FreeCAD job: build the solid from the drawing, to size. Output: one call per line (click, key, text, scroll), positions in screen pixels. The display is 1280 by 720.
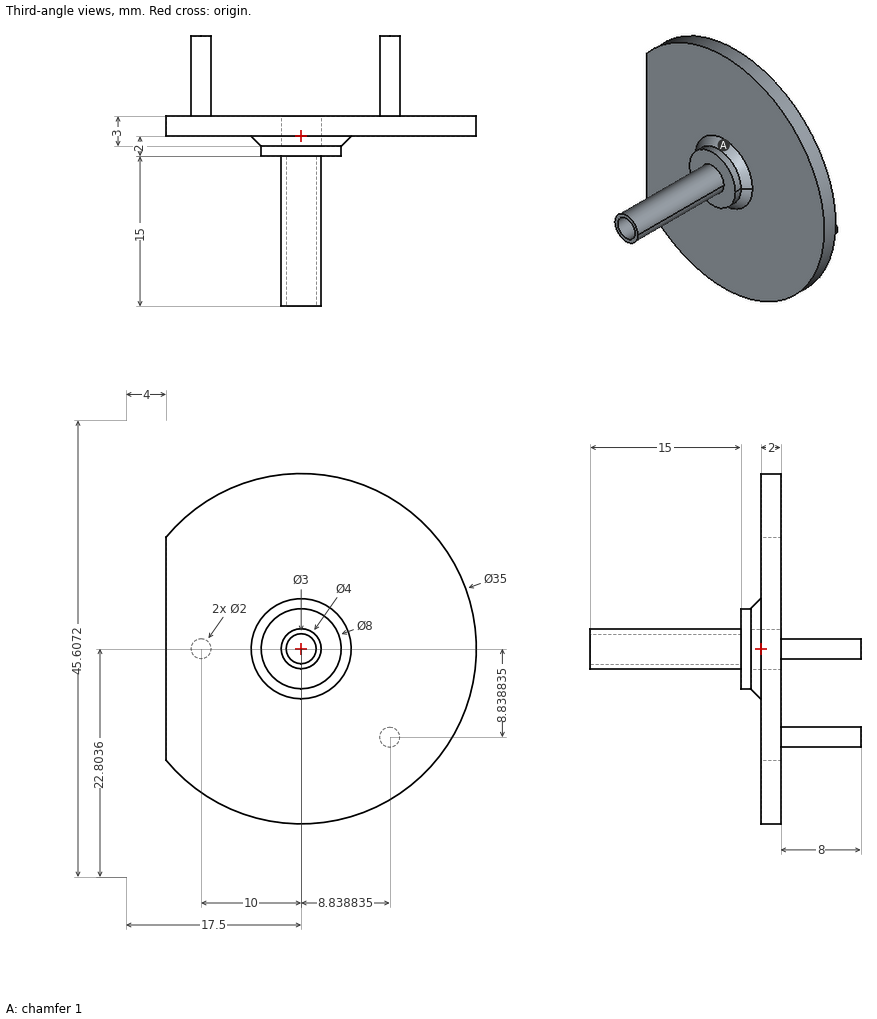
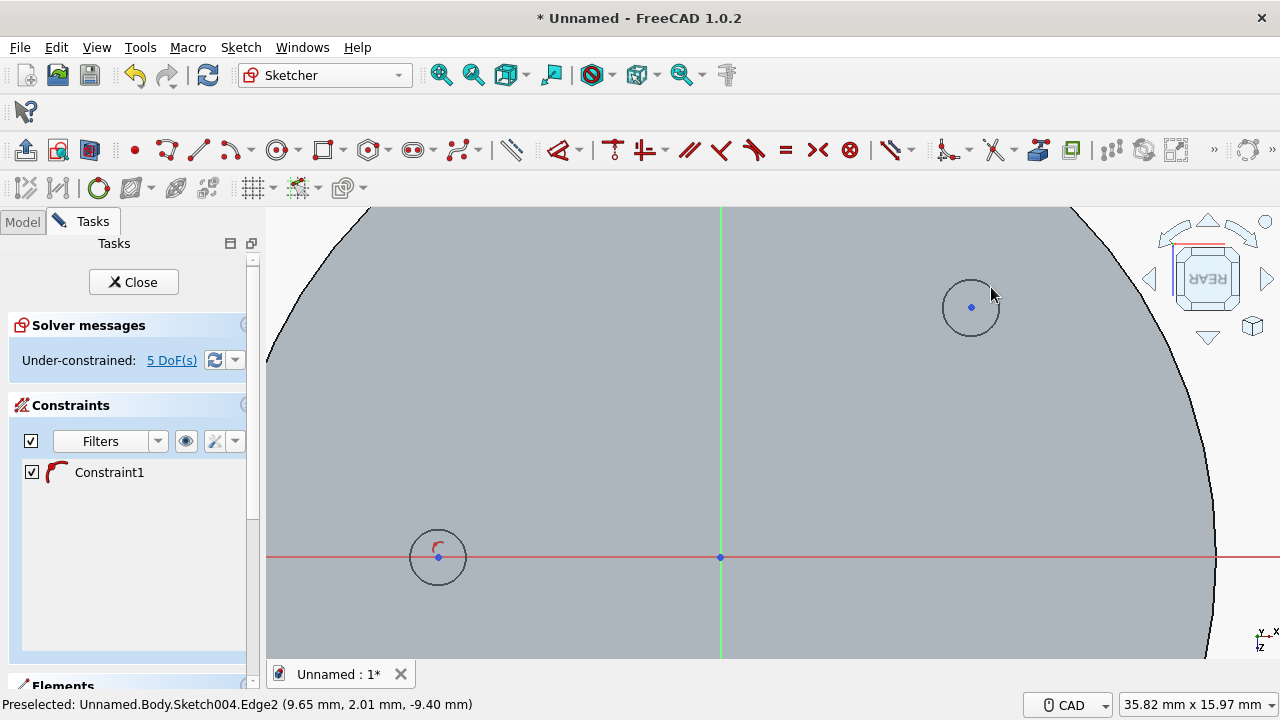
click(458, 538)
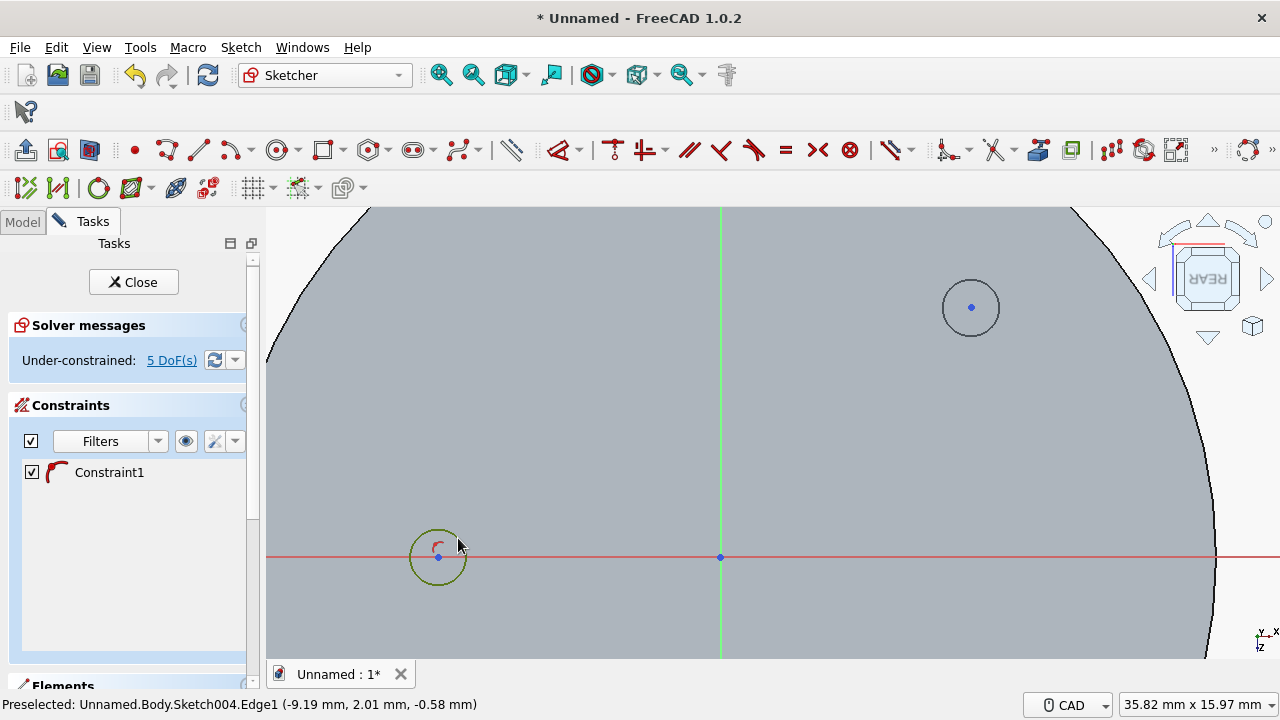
click(991, 288)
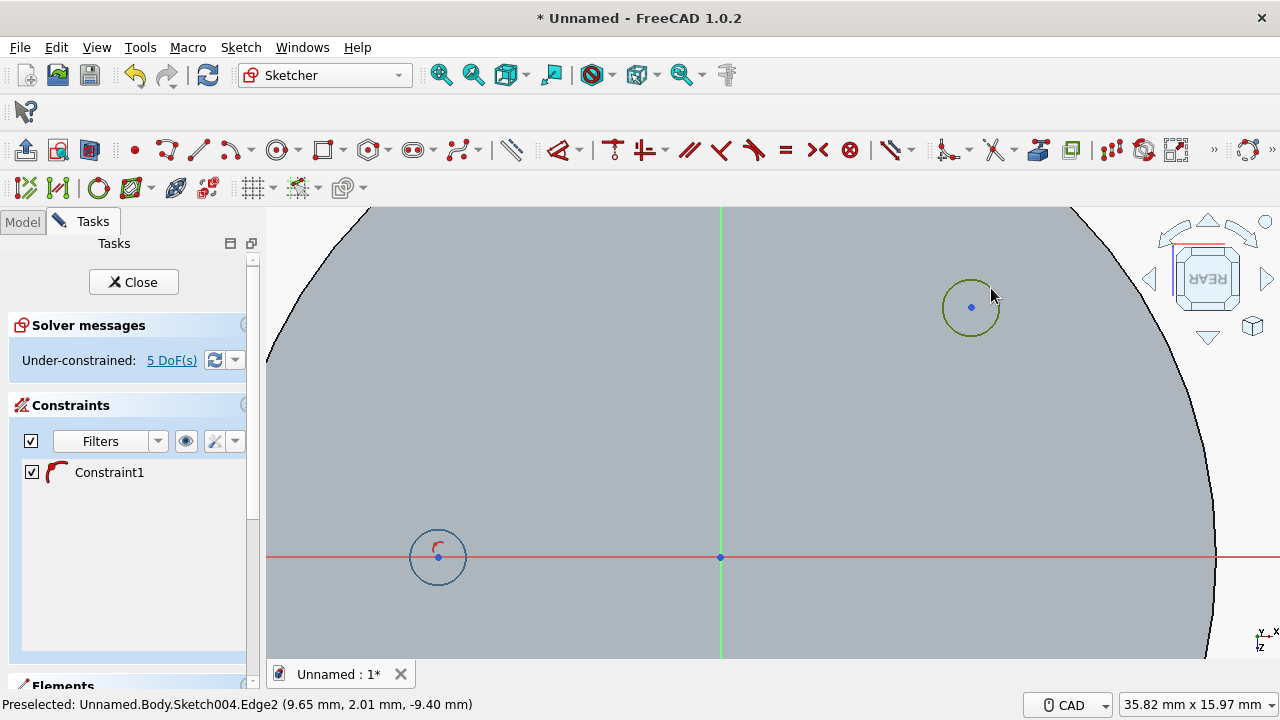
click(786, 150)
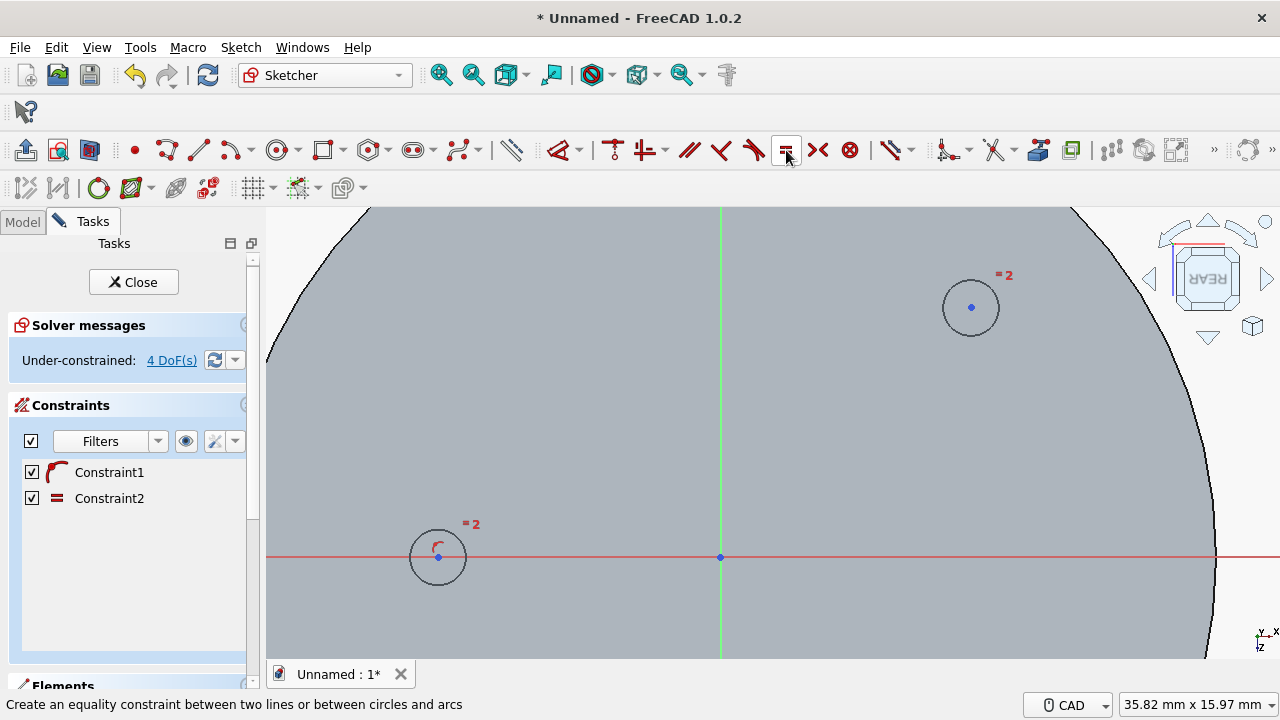
click(558, 150)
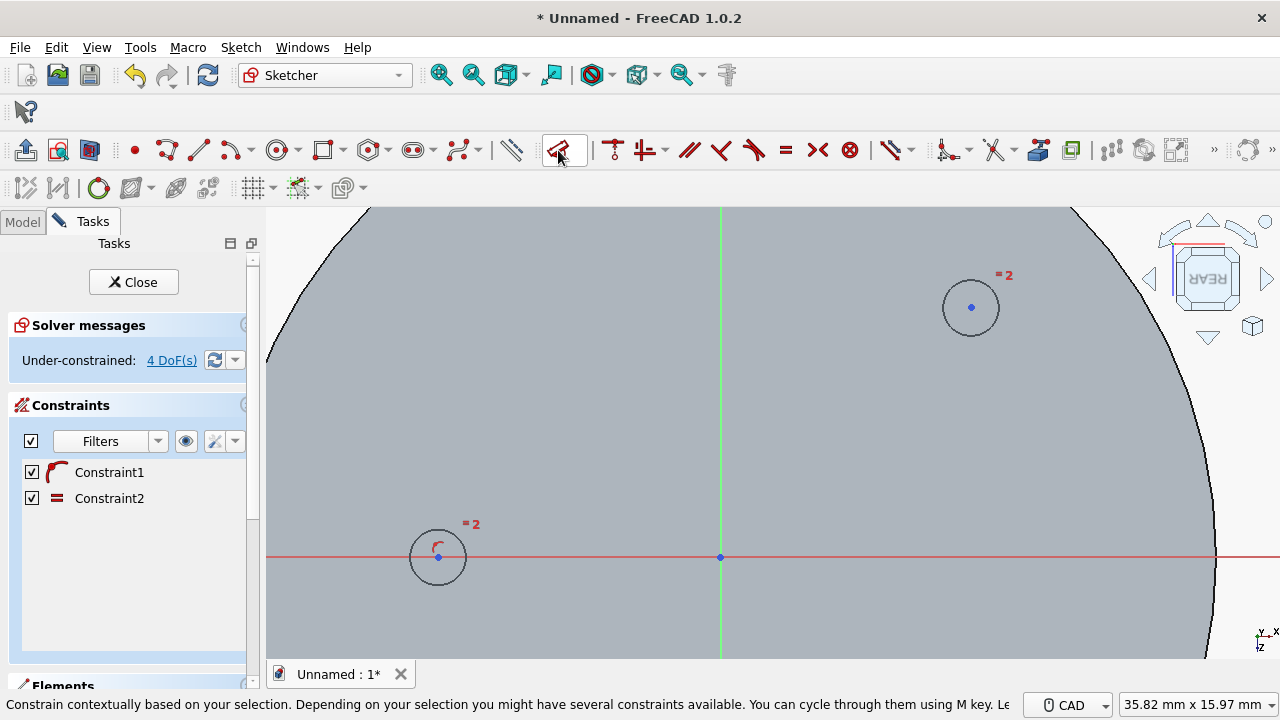
click(458, 538)
click(481, 516)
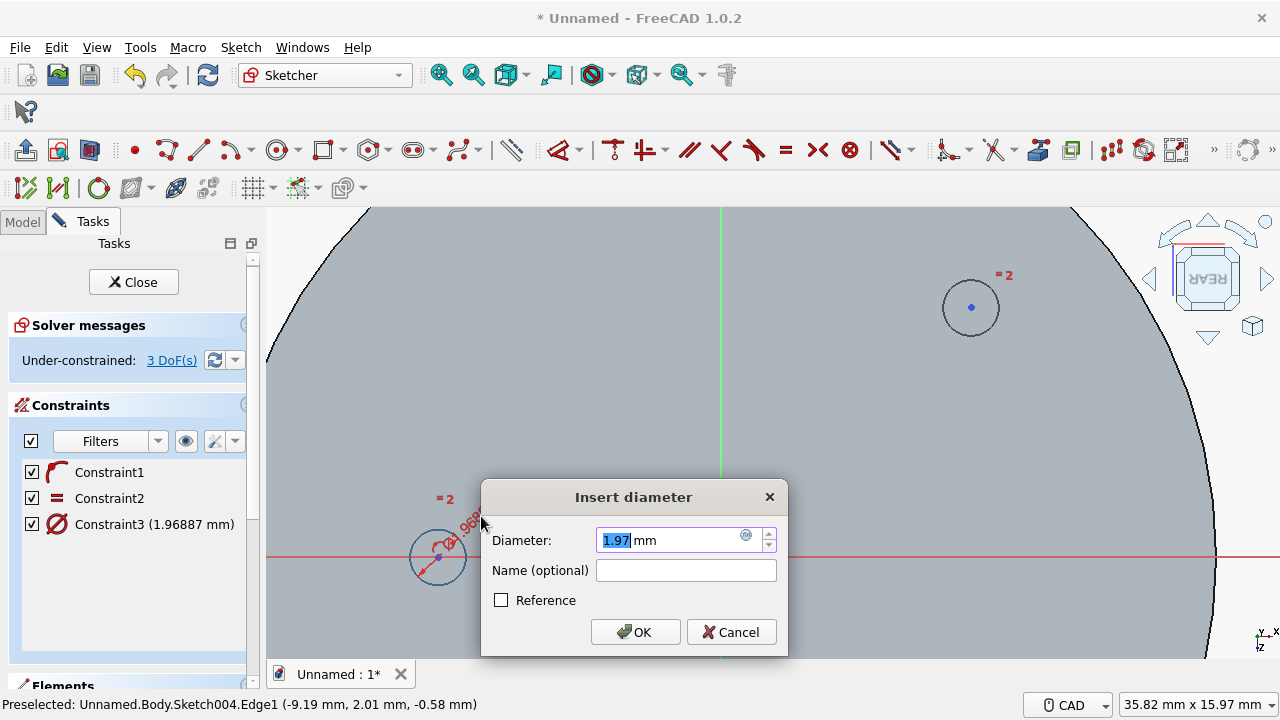
text(2)
key(Return)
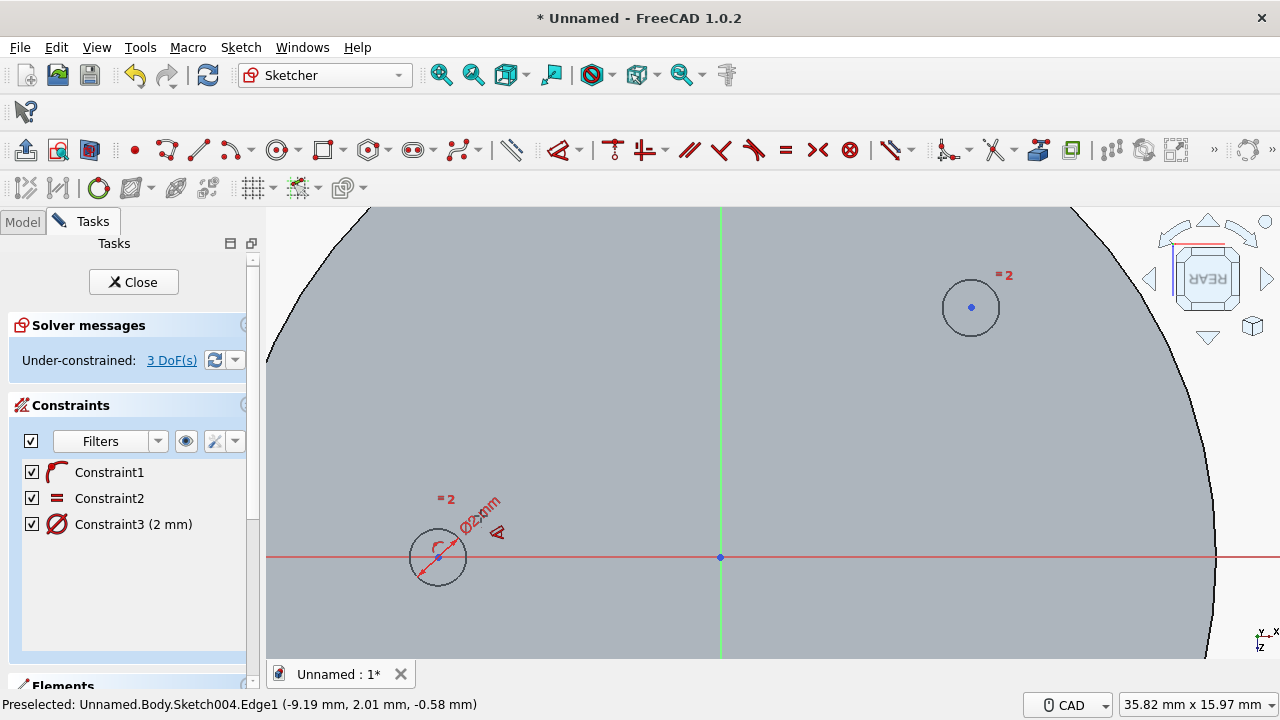
click(438, 557)
click(579, 591)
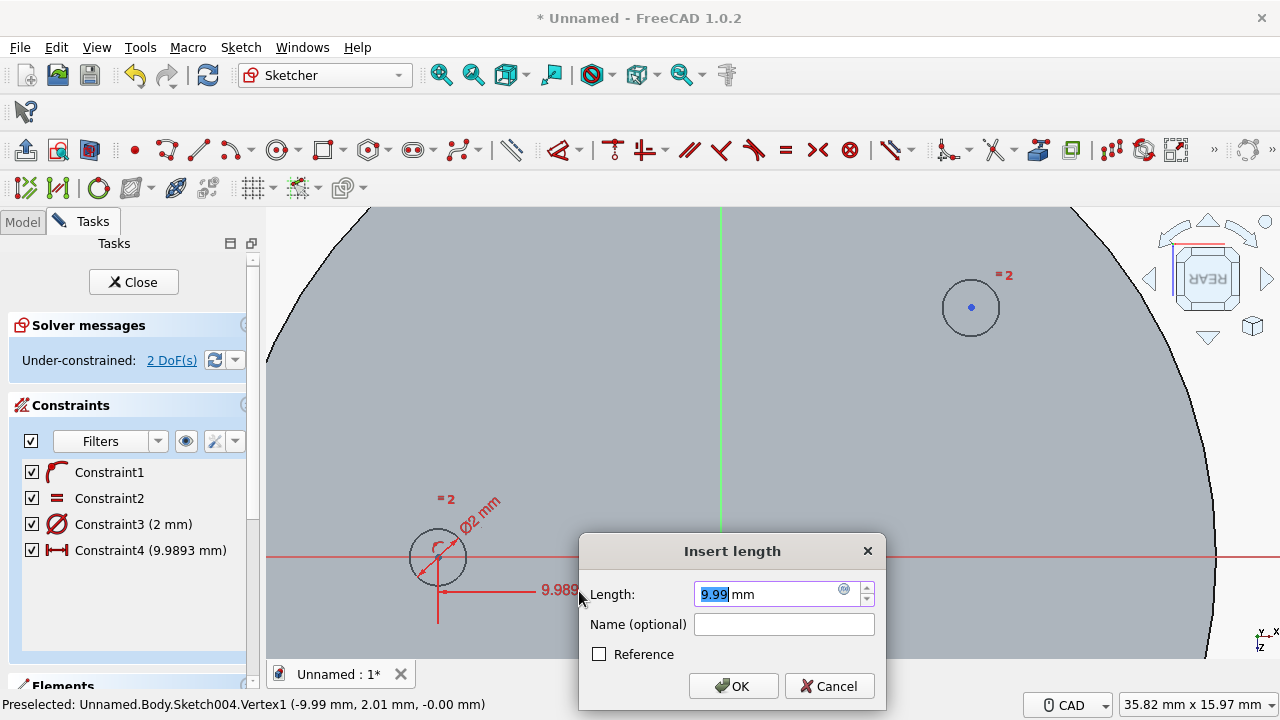
text(10)
key(Return)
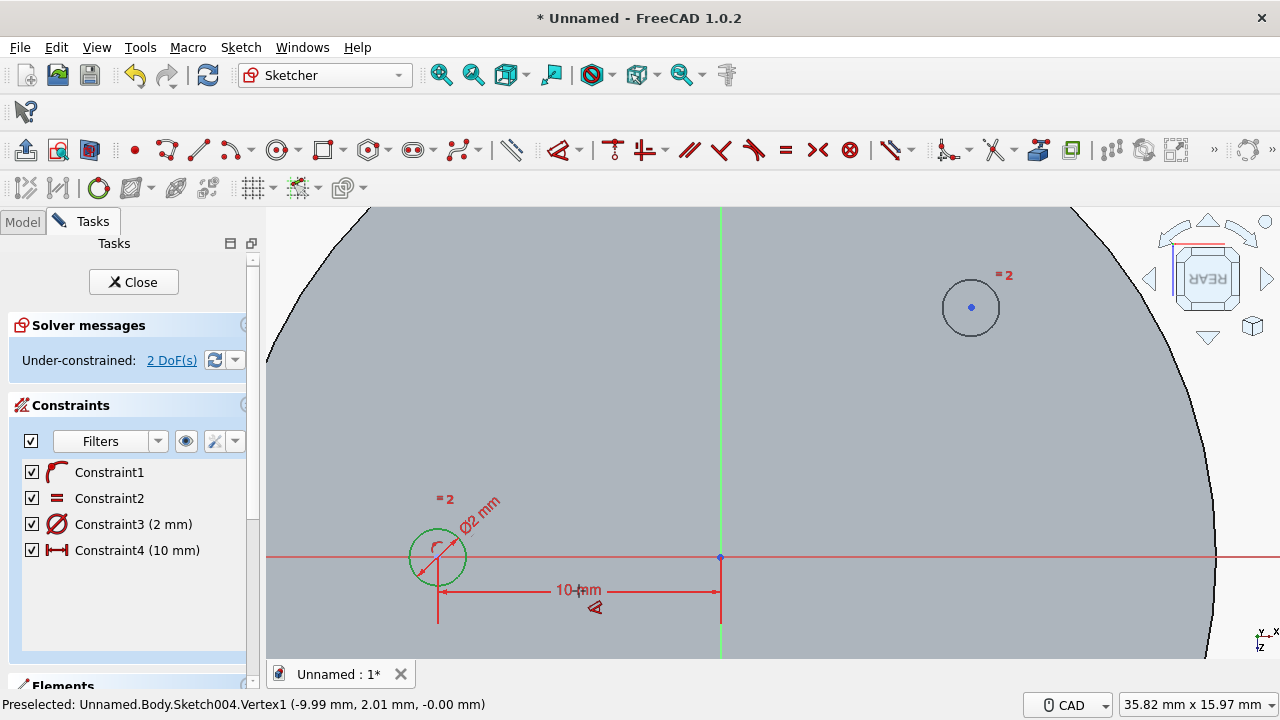
click(971, 308)
click(846, 591)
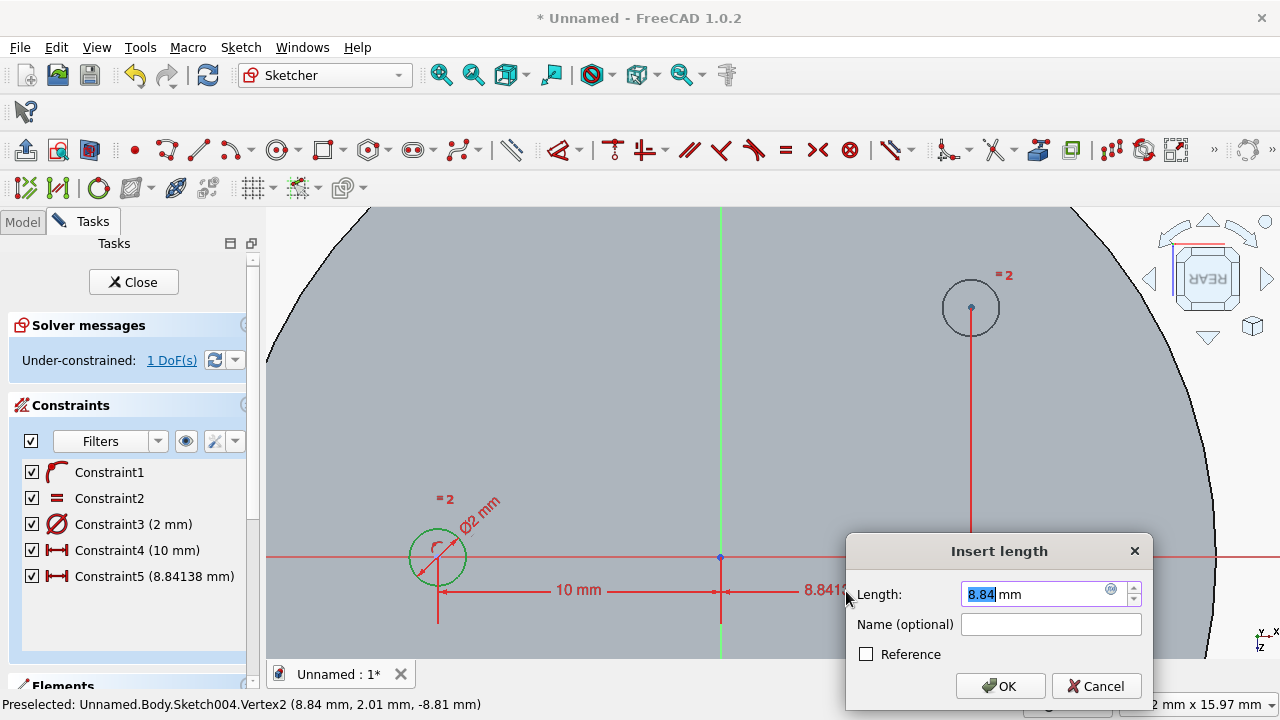
text(8.838835)
key(Return)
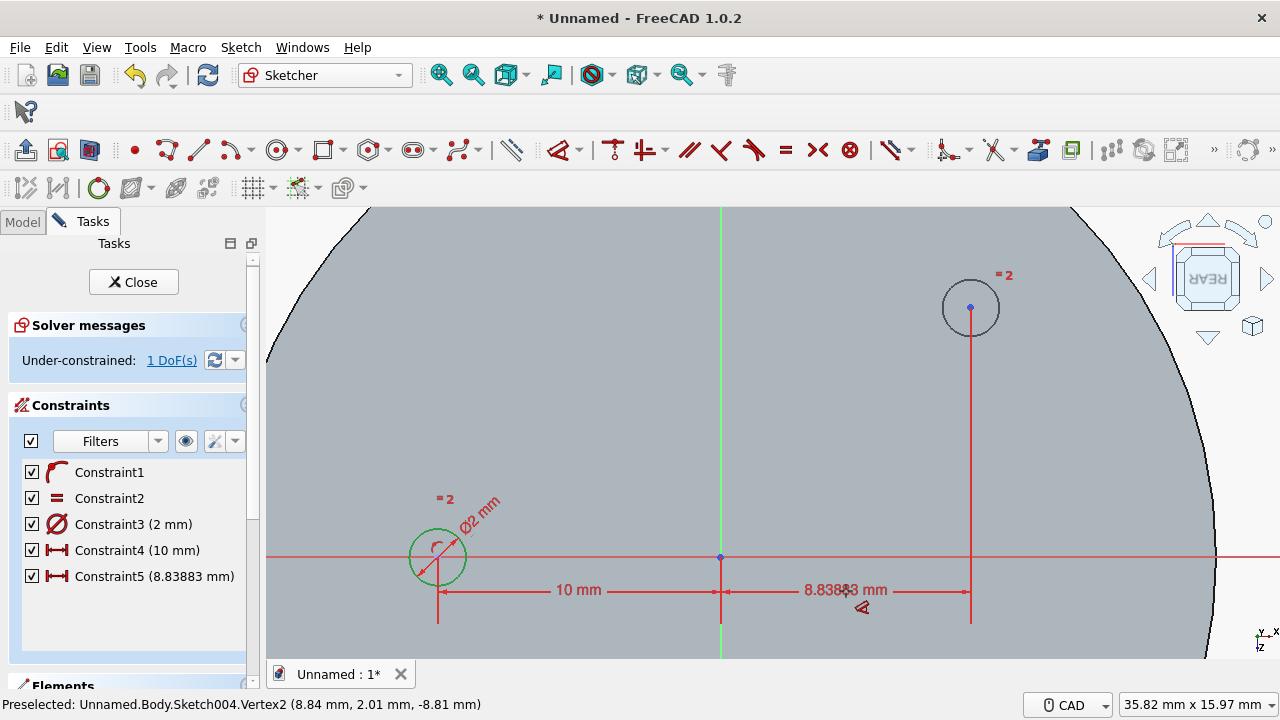
click(971, 308)
click(1005, 433)